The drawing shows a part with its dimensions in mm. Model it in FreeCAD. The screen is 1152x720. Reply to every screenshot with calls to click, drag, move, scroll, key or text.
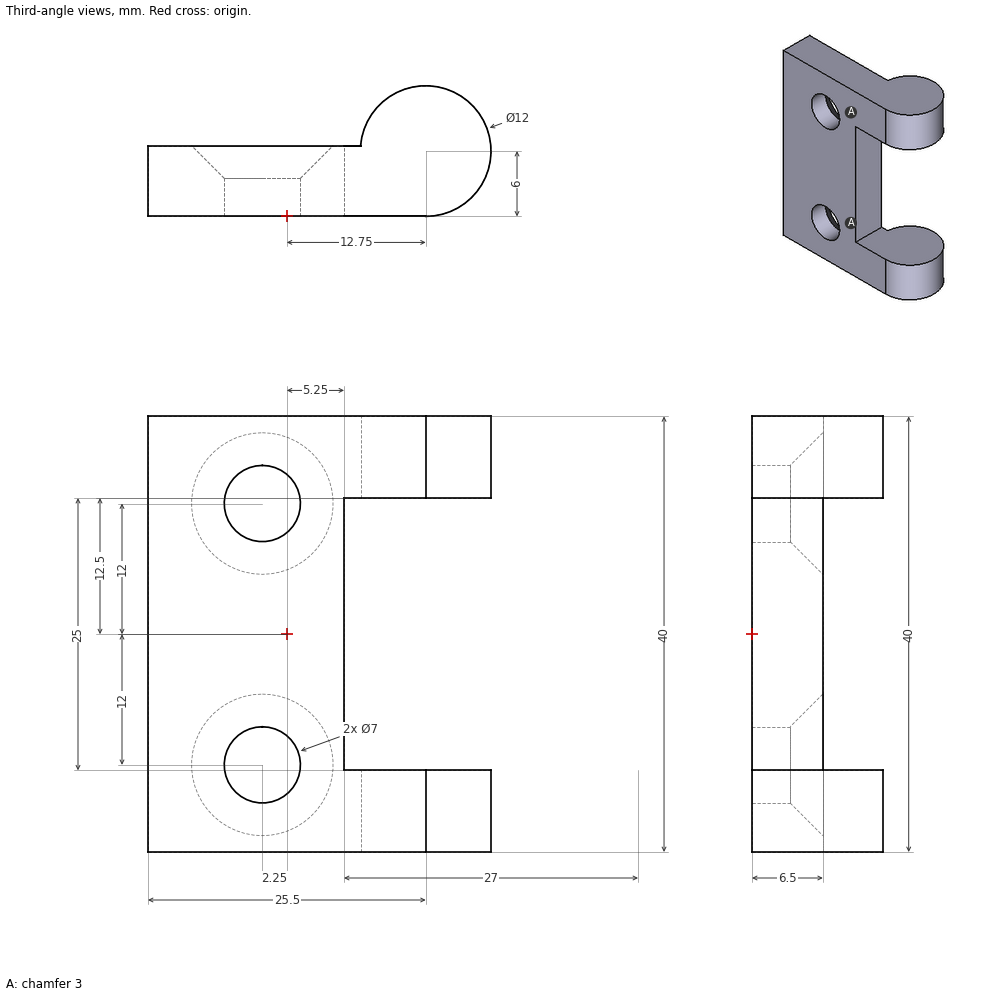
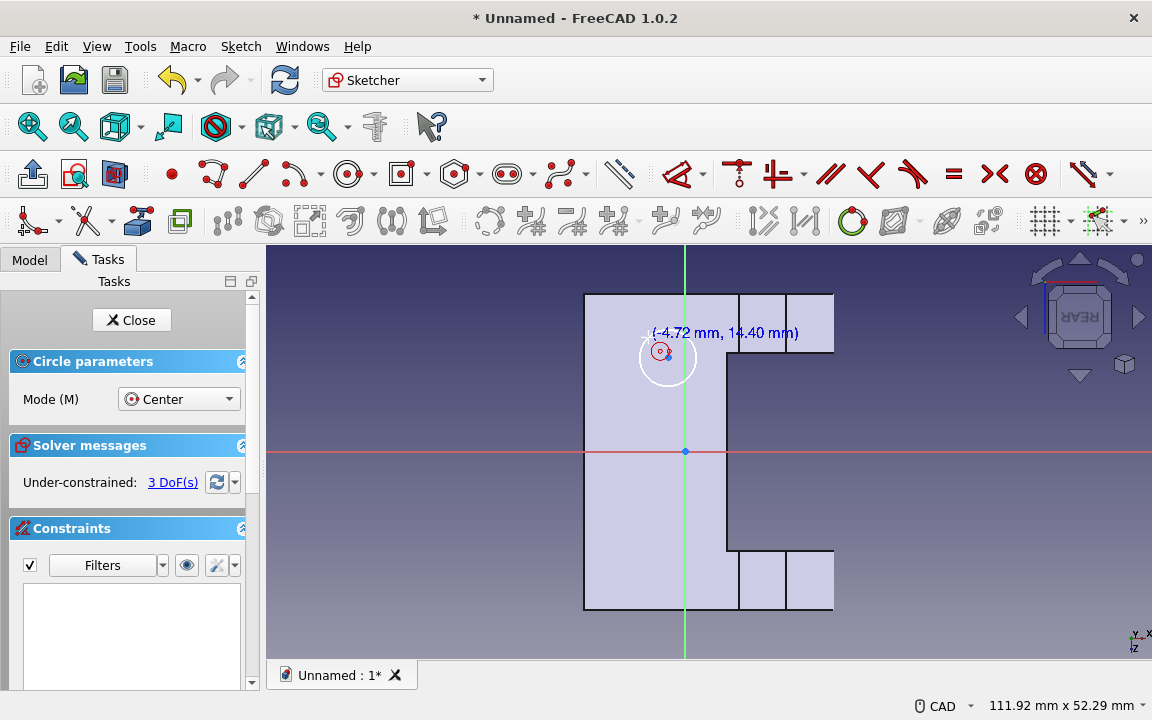
click(668, 547)
click(648, 527)
key(Escape)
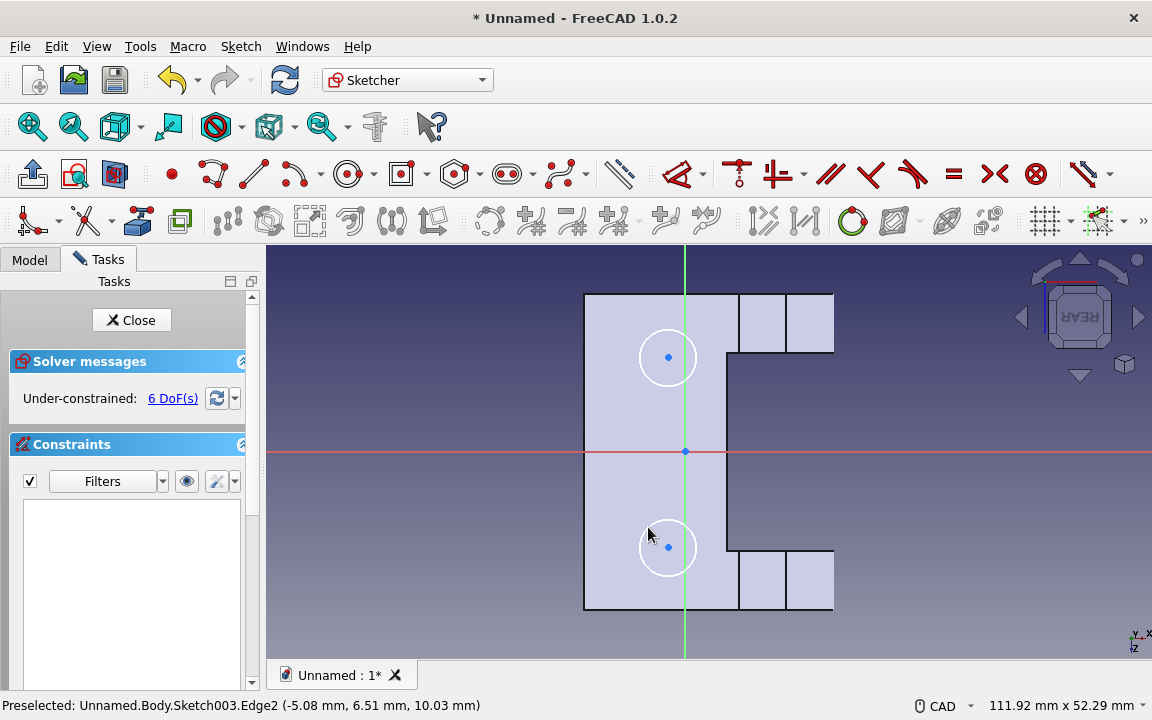
click(688, 338)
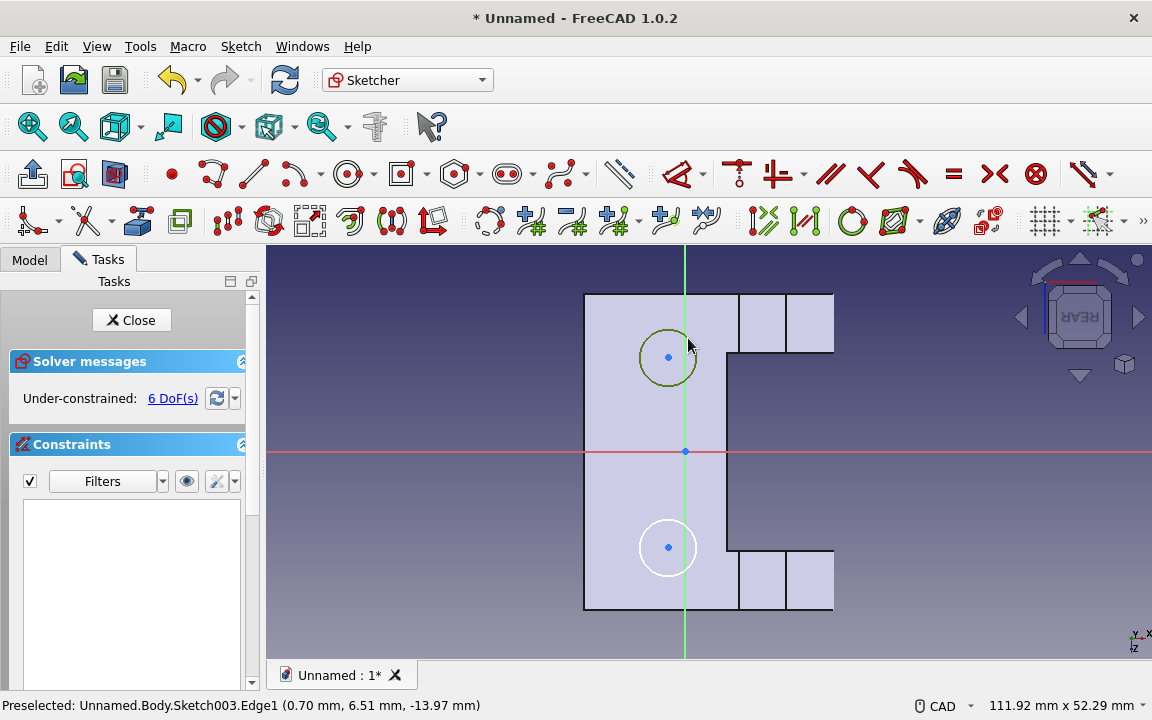
click(688, 528)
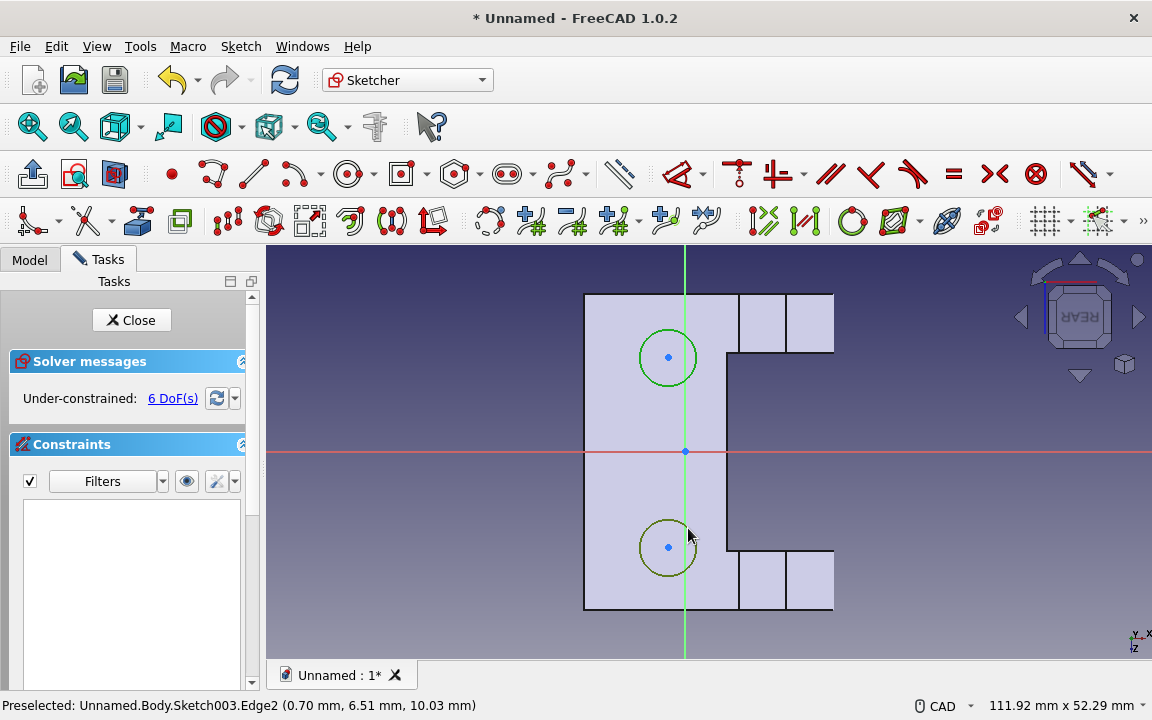
click(954, 174)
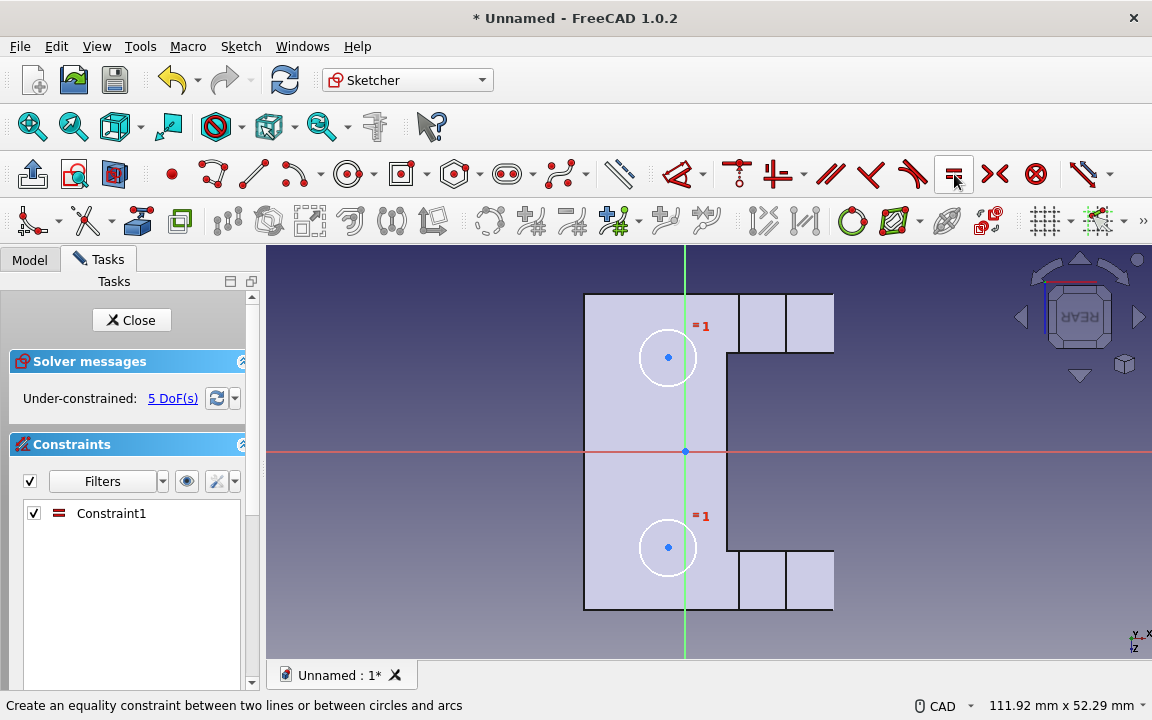
click(668, 358)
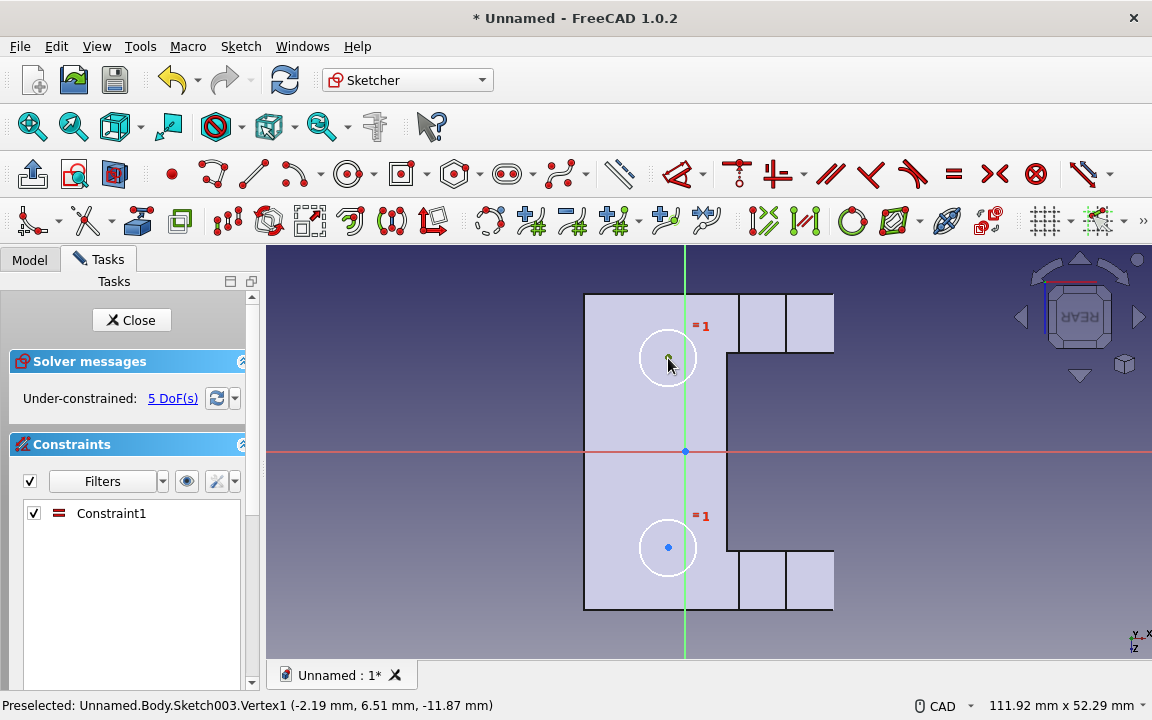
click(668, 548)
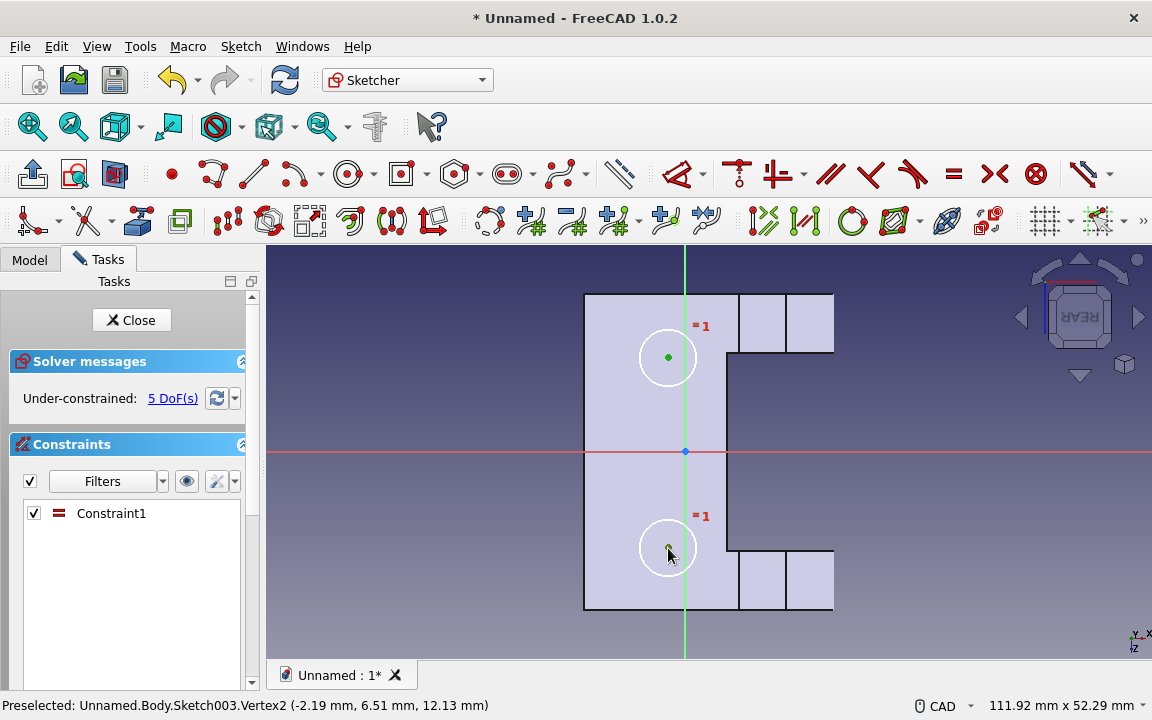
click(804, 174)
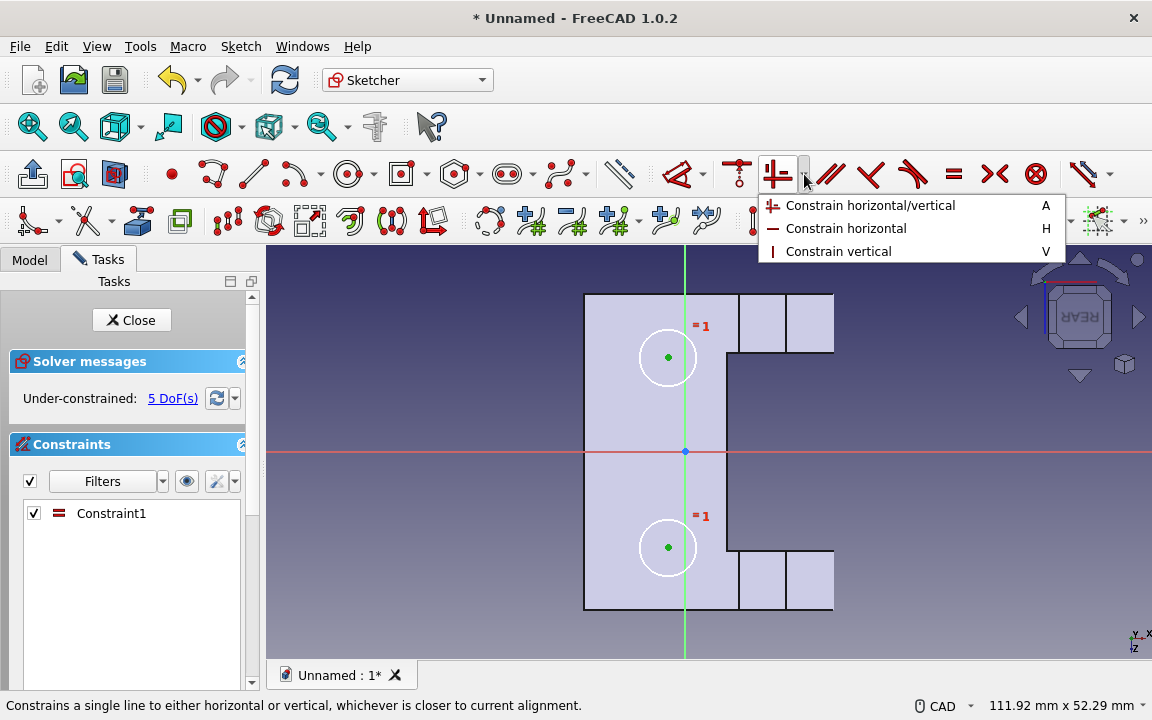
click(912, 252)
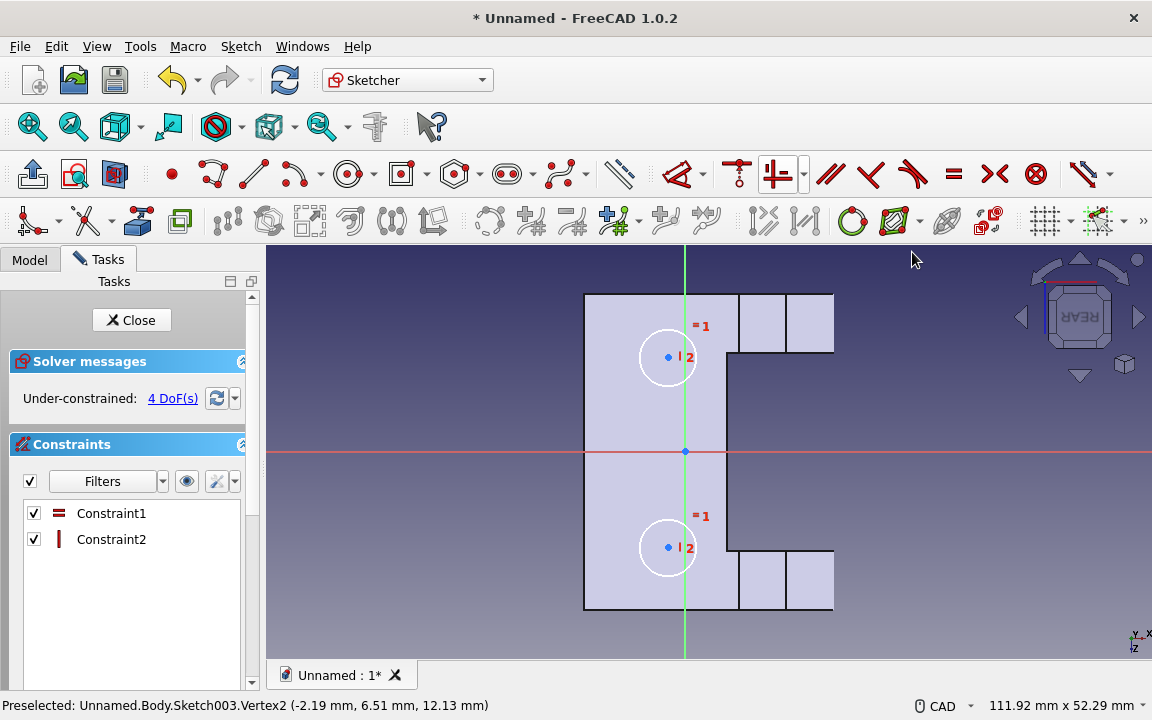
click(676, 174)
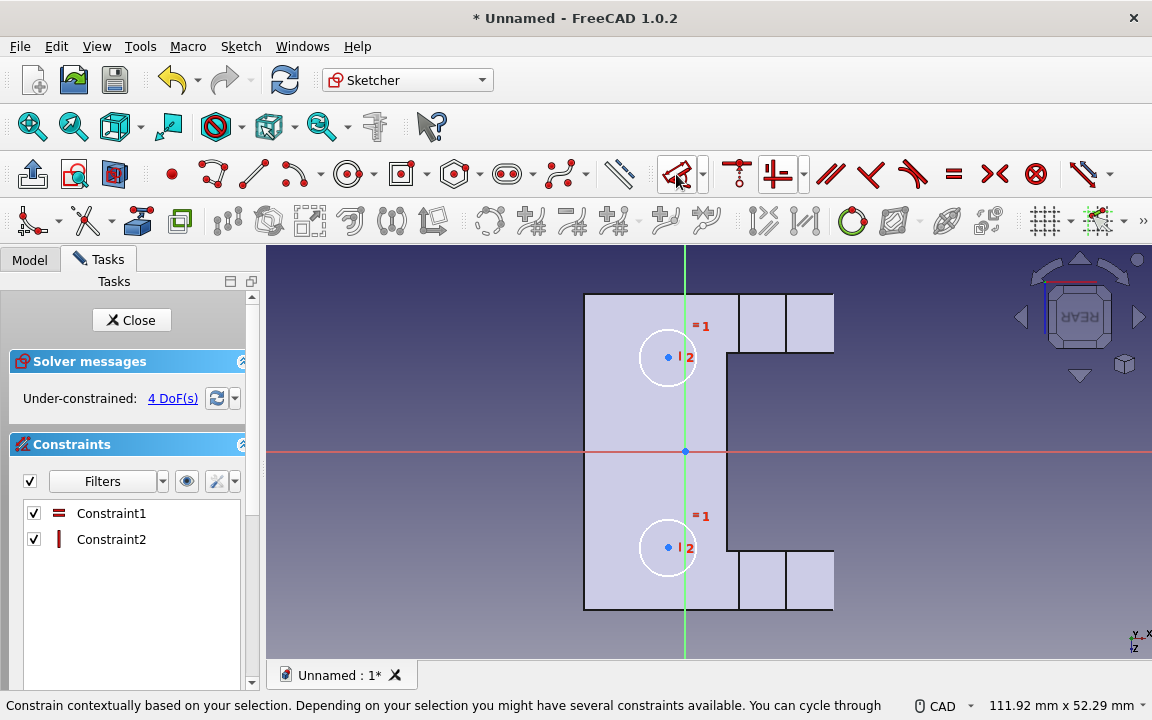
click(688, 338)
click(711, 315)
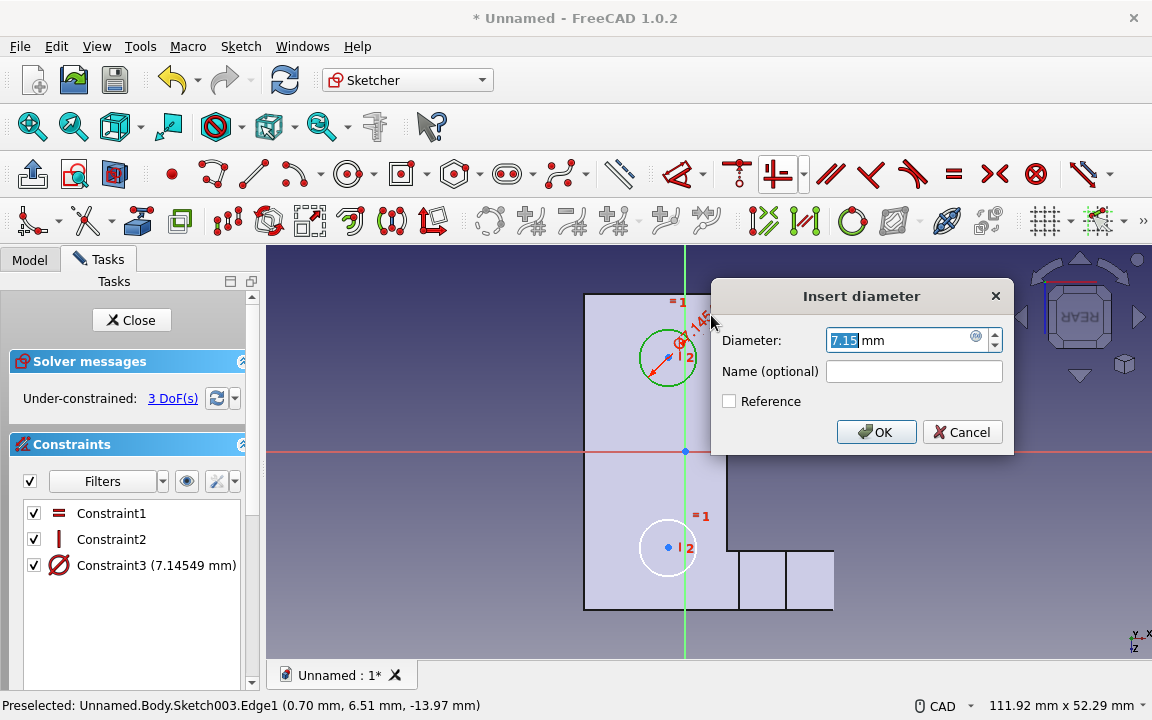
text(7)
key(Return)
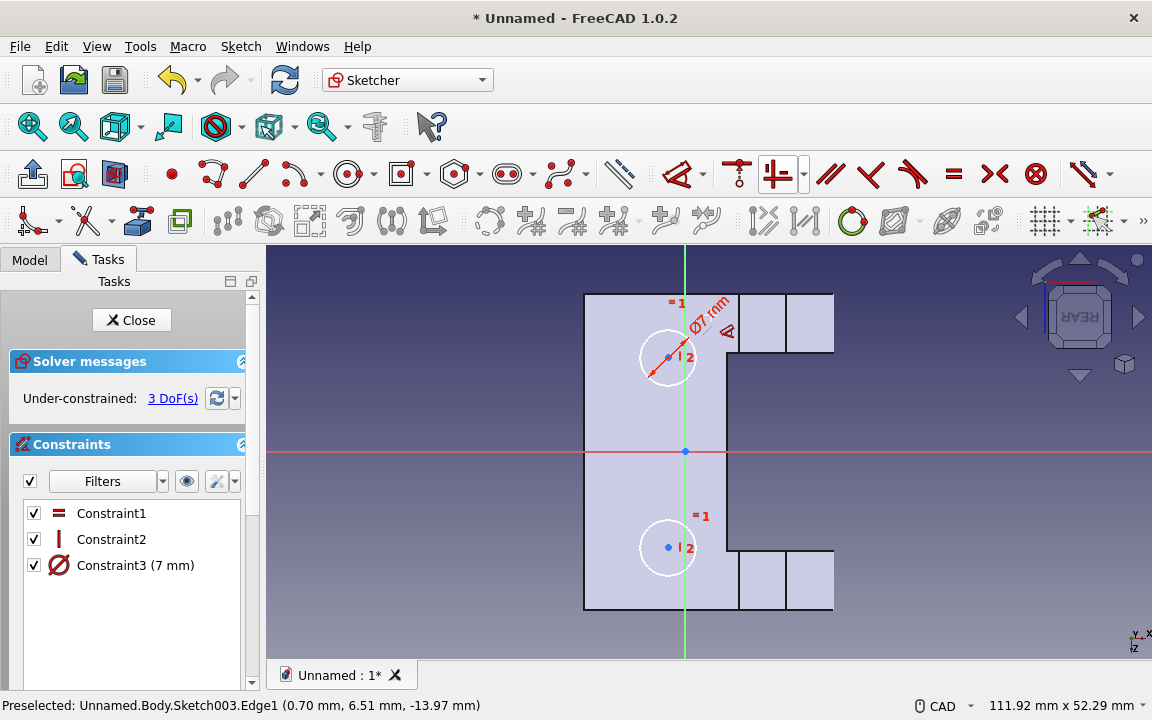
click(668, 358)
click(719, 405)